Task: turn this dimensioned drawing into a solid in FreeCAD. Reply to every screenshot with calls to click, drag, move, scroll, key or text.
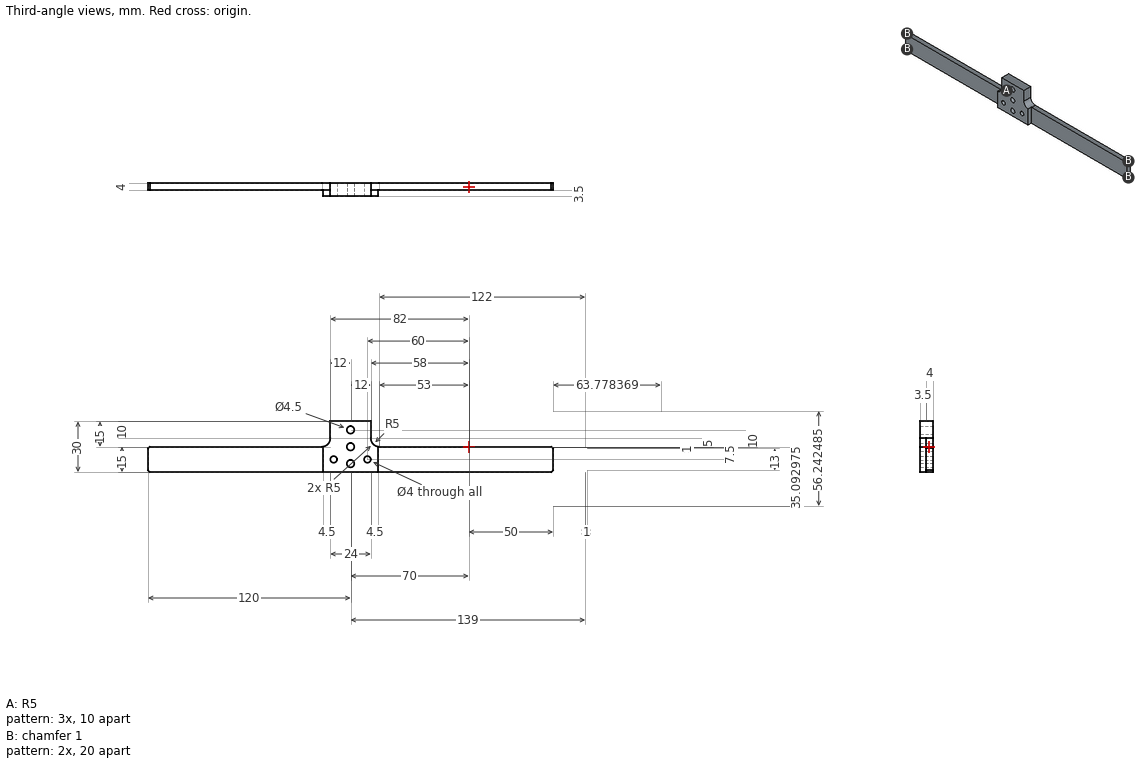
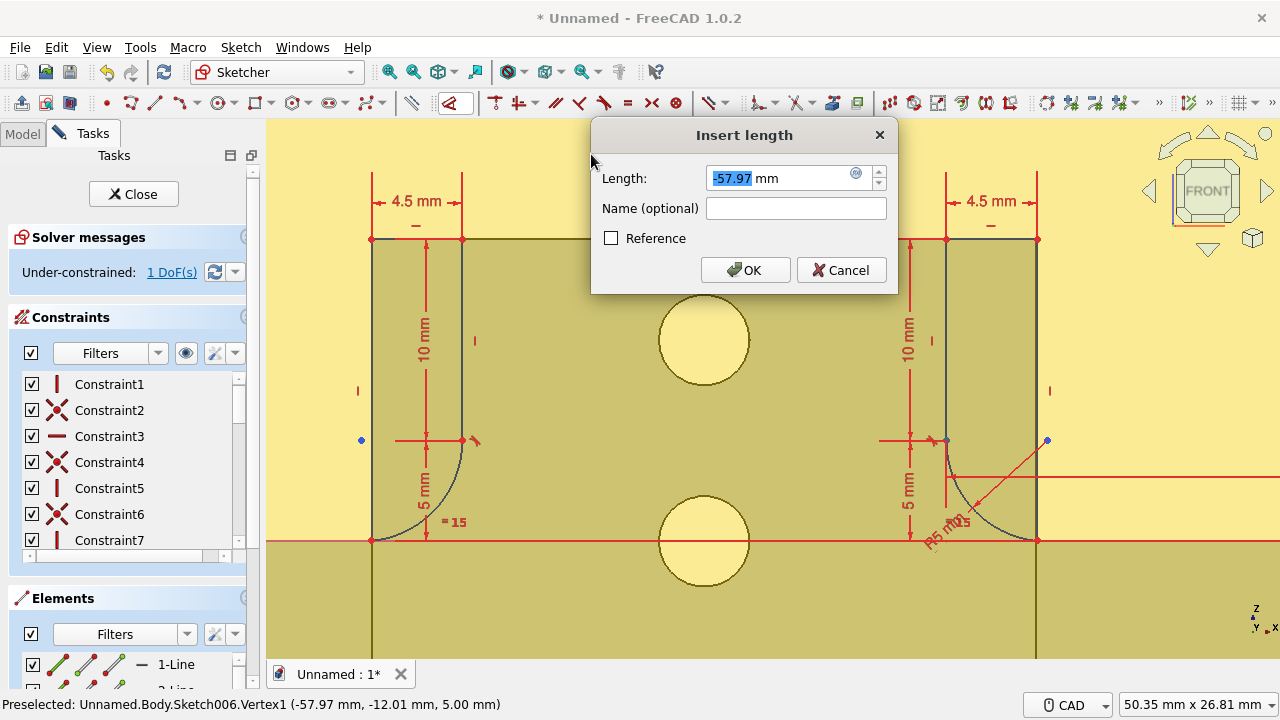
text(-58)
key(Return)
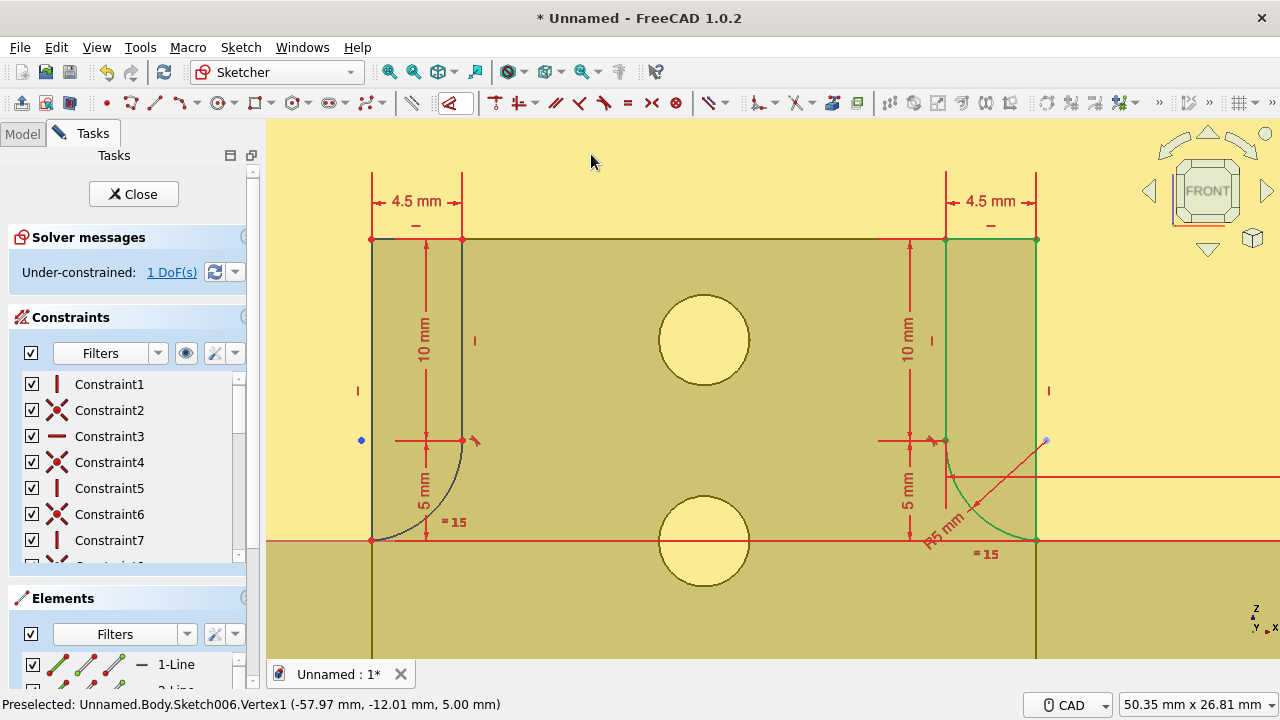
click(462, 239)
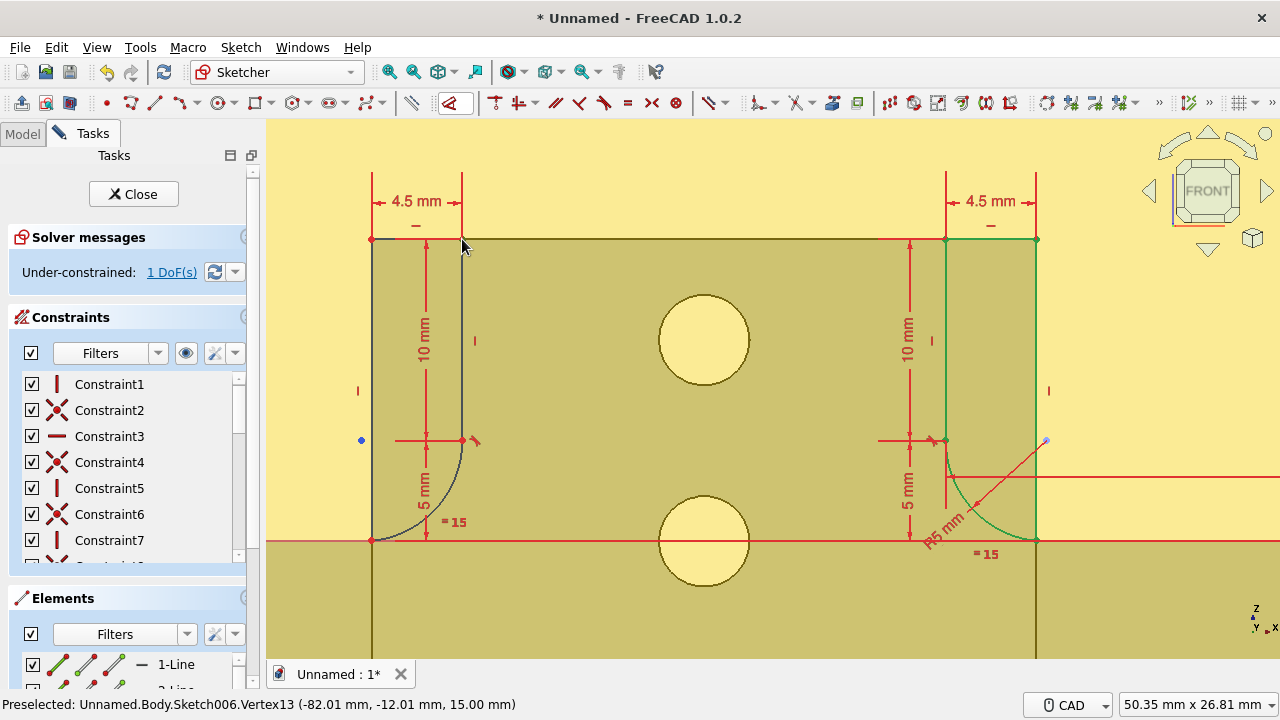
click(468, 104)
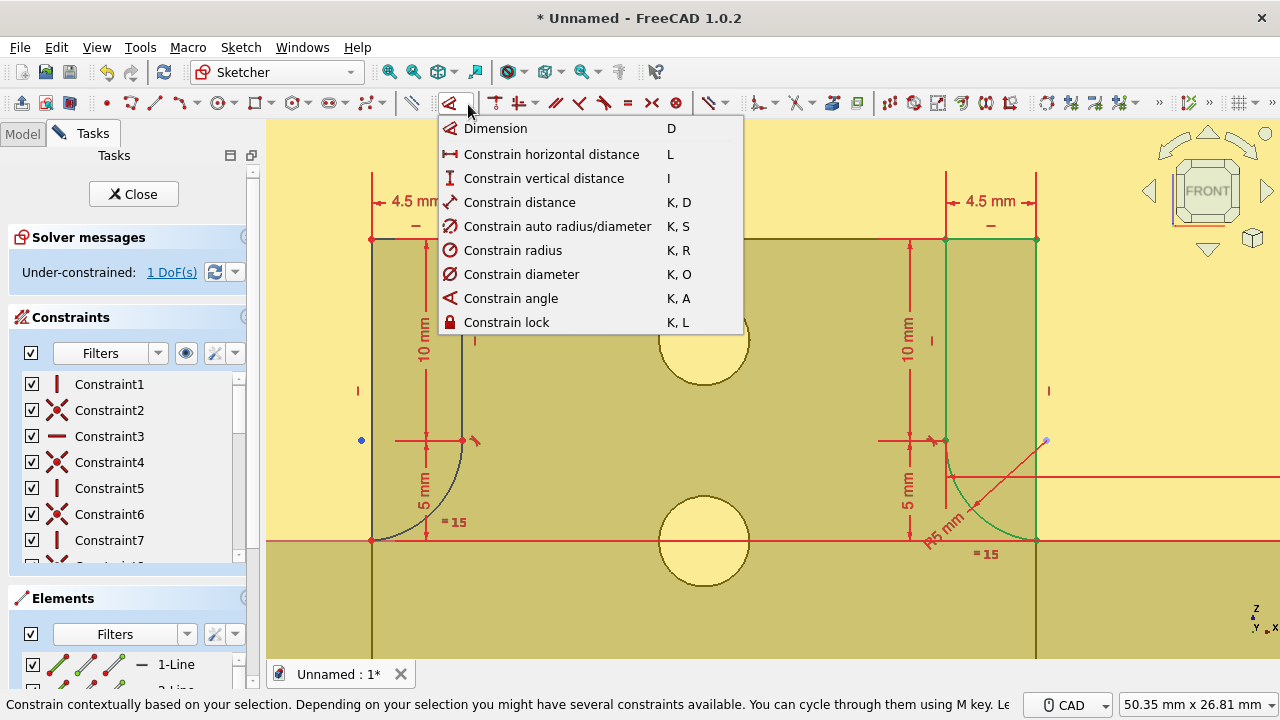
click(591, 154)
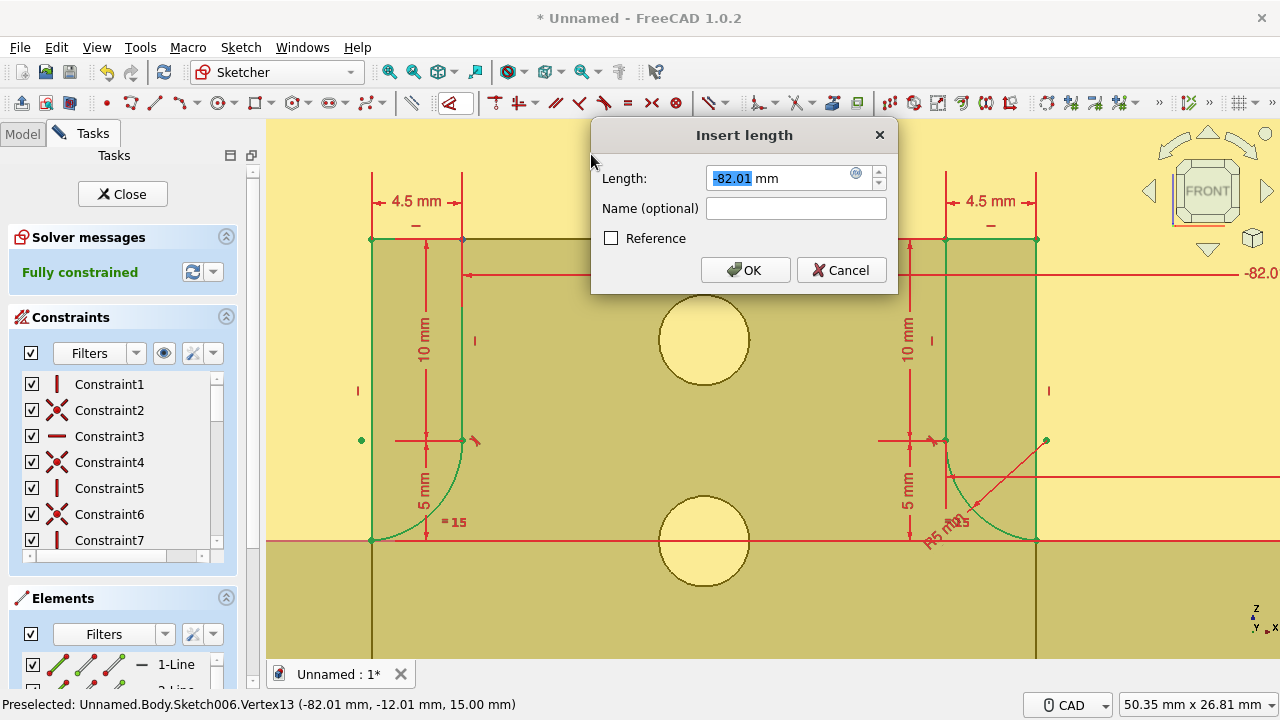
text(-82)
key(Return)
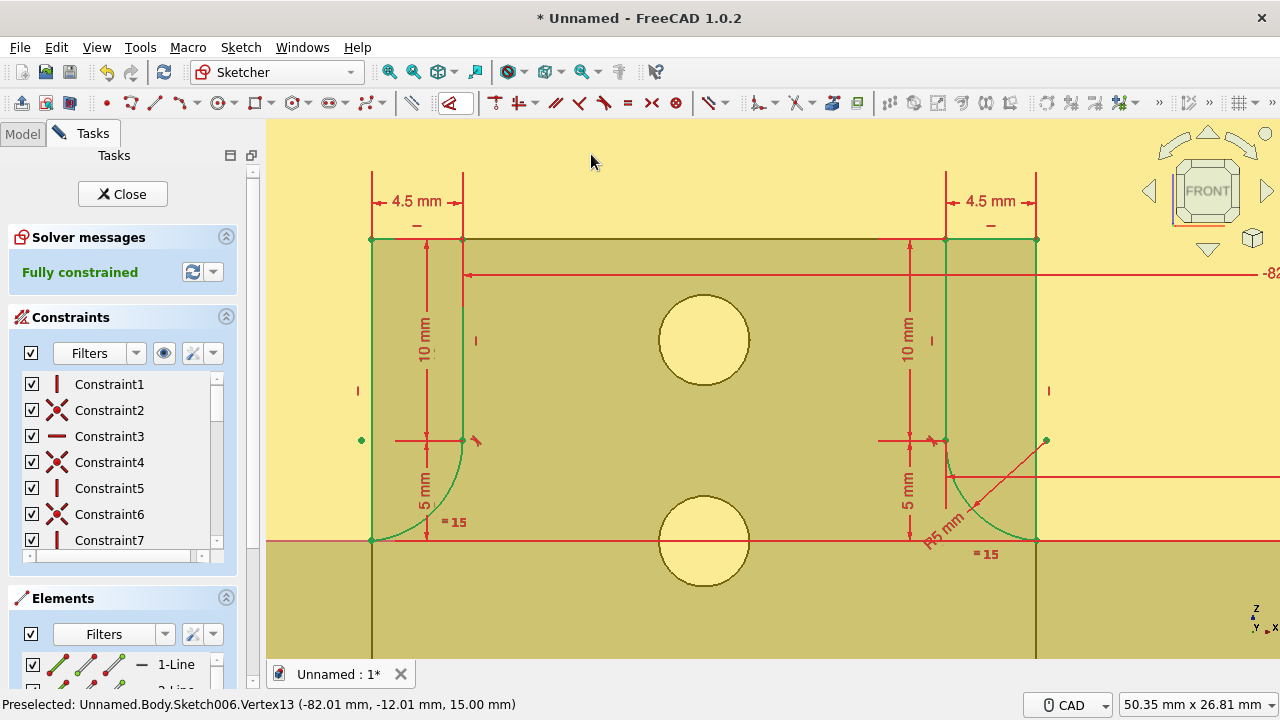
click(123, 194)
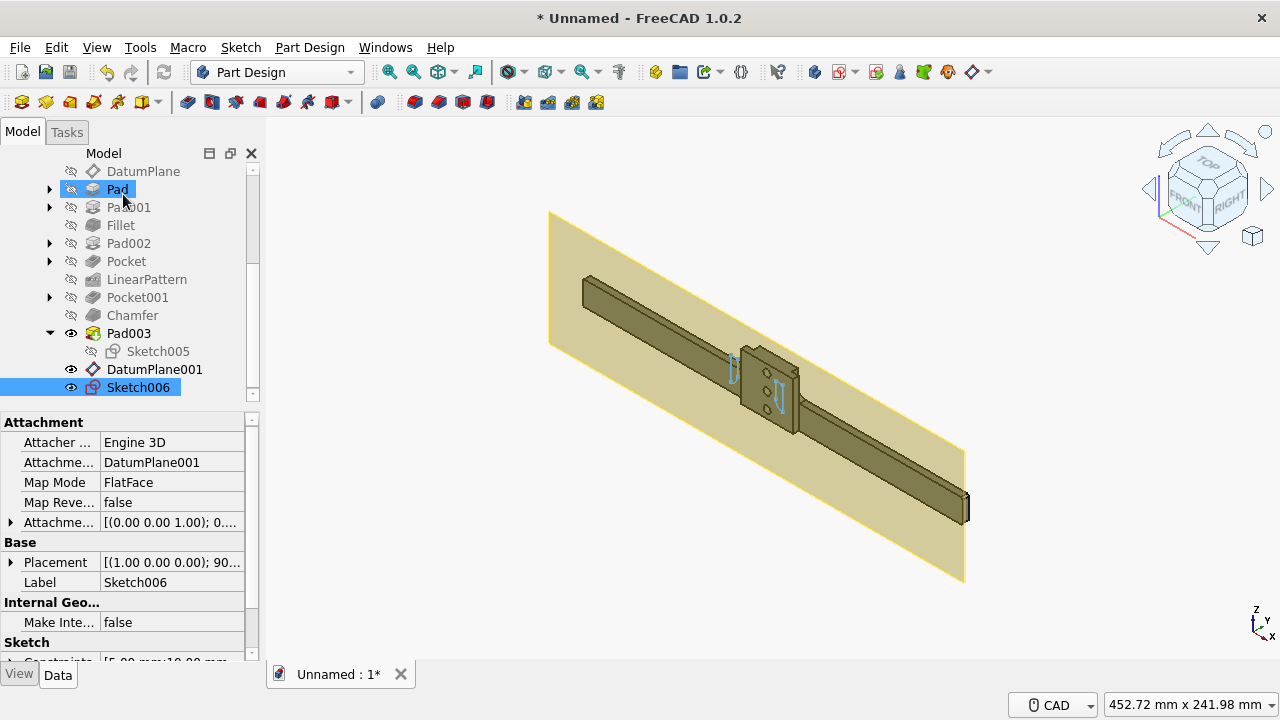
click(188, 102)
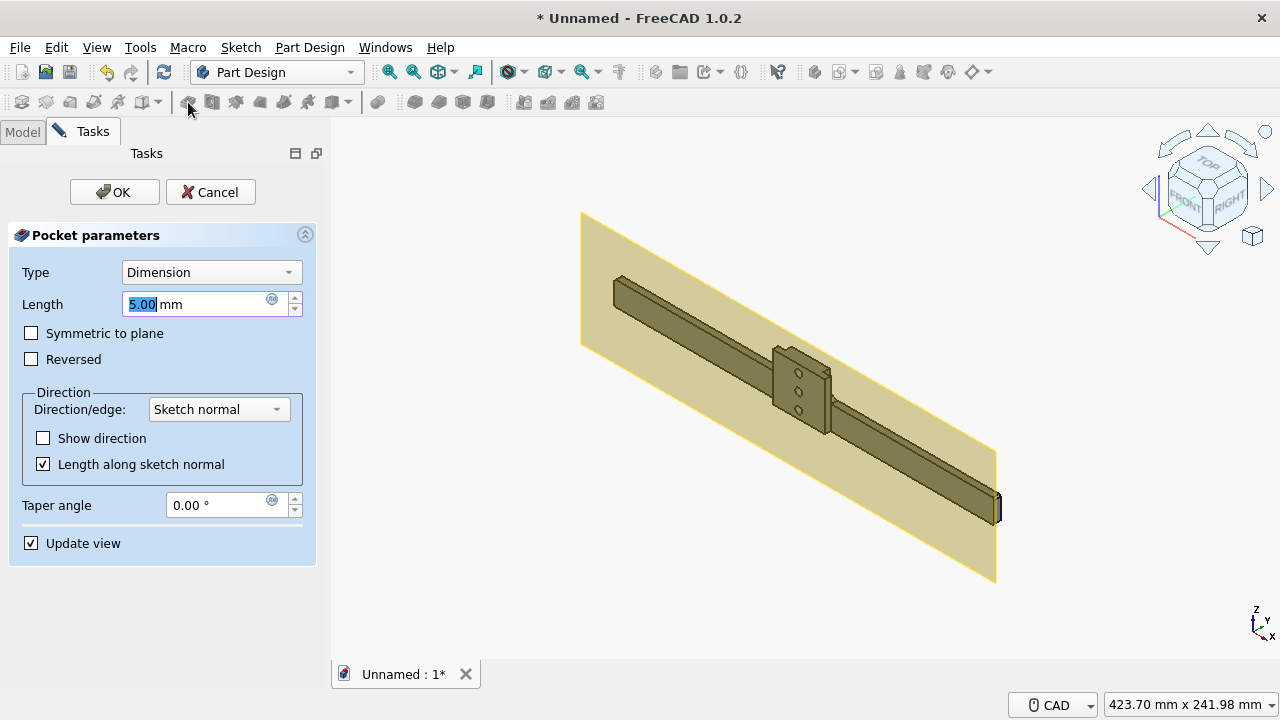
text(10)
key(Tab)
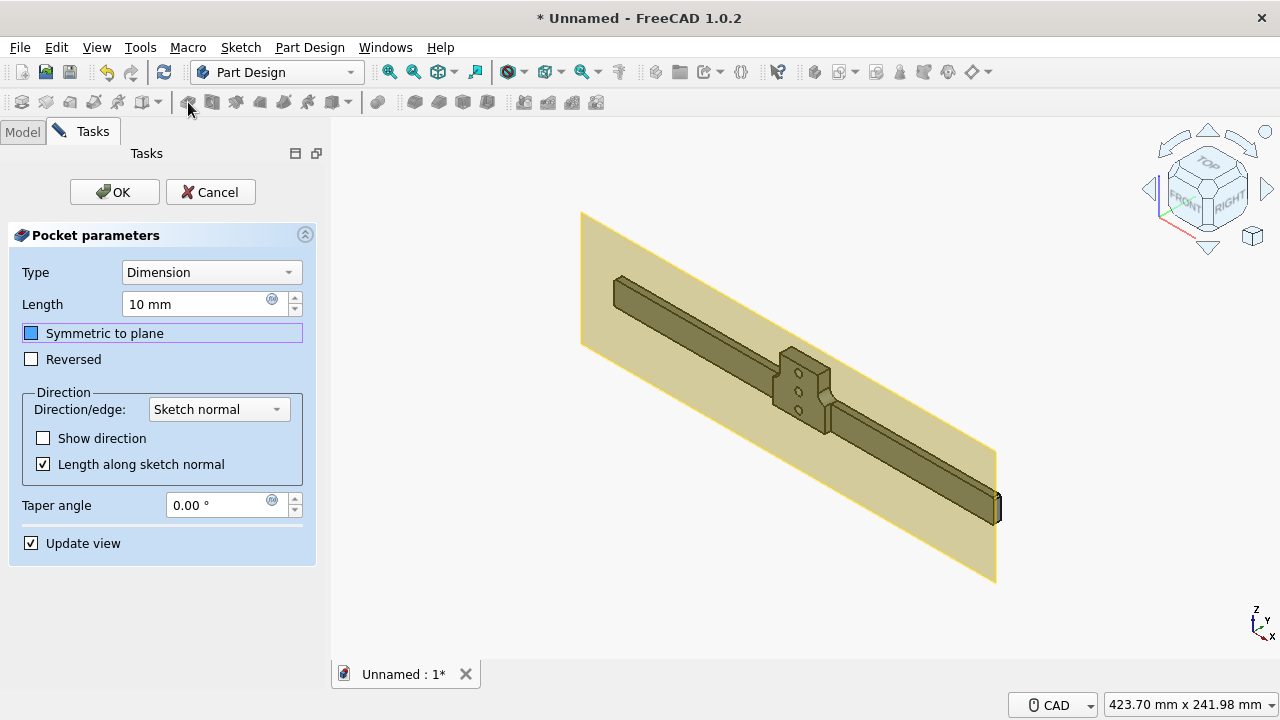
click(115, 192)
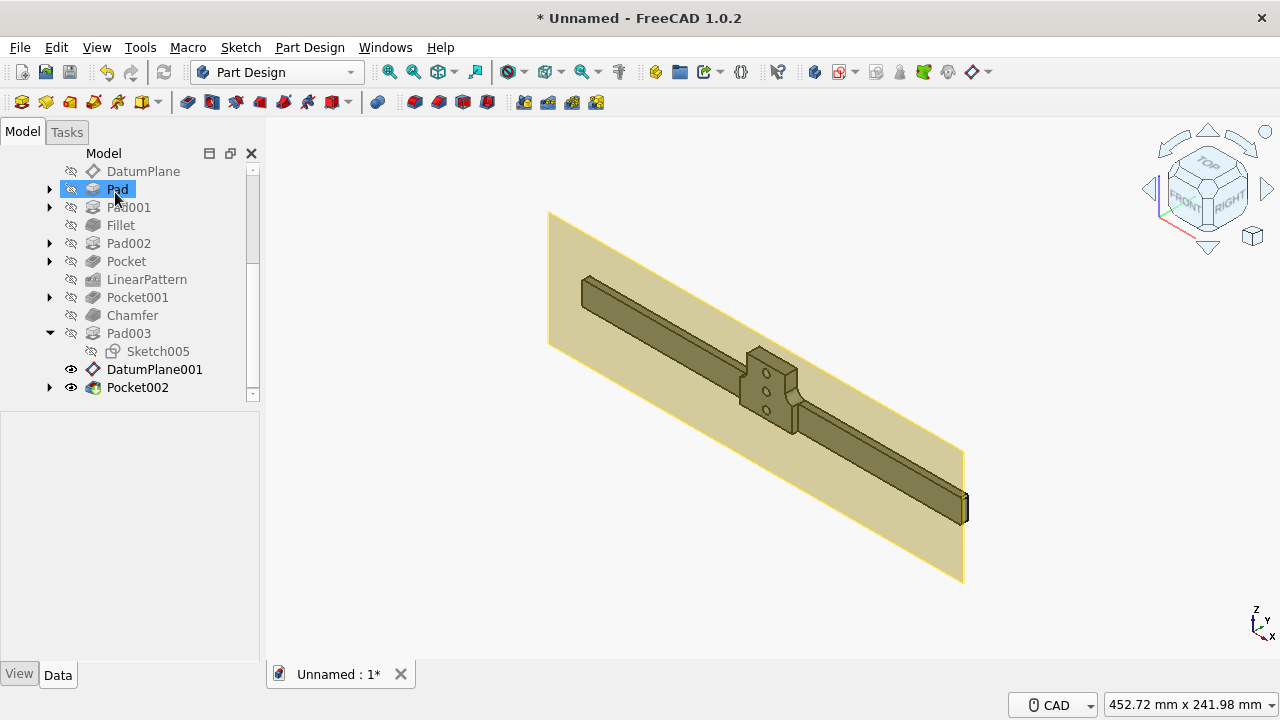
click(116, 369)
key(space)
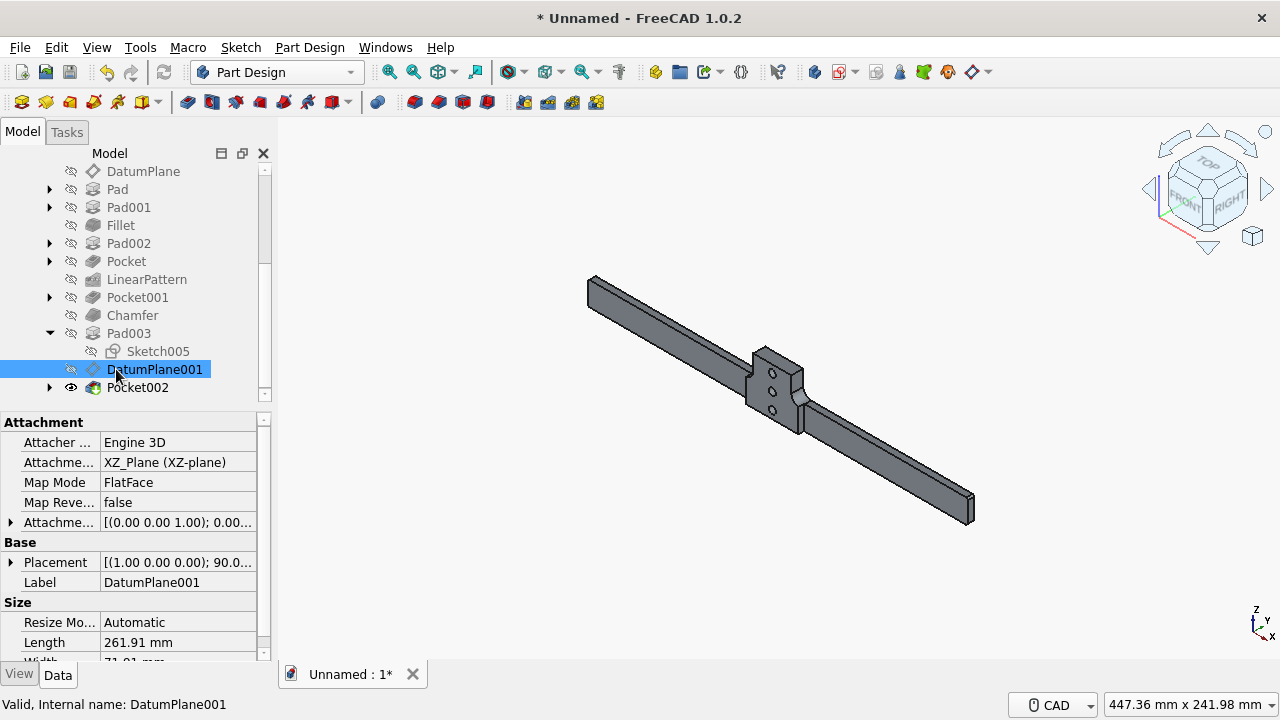
key(4)